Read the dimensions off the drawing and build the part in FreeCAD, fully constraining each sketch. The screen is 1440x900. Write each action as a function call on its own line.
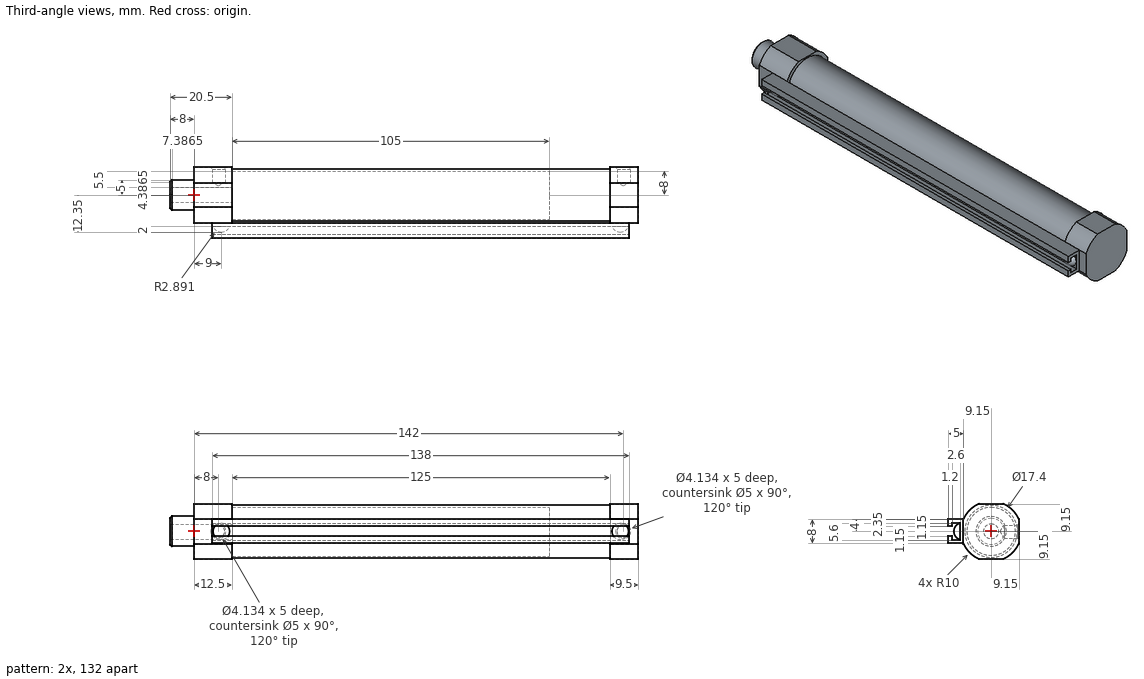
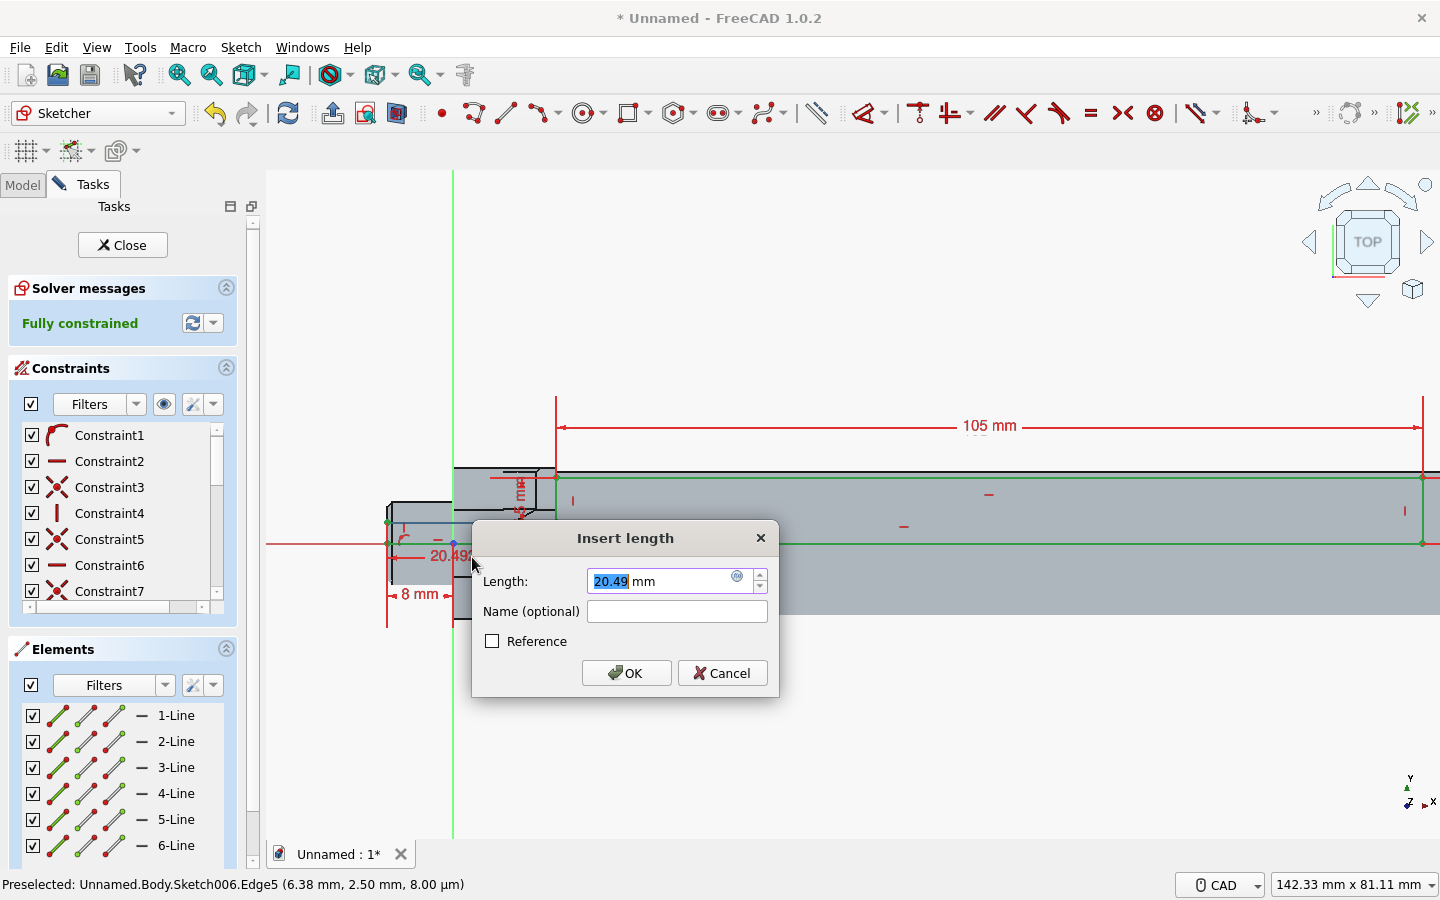
text(20.5)
key(Return)
key(Escape)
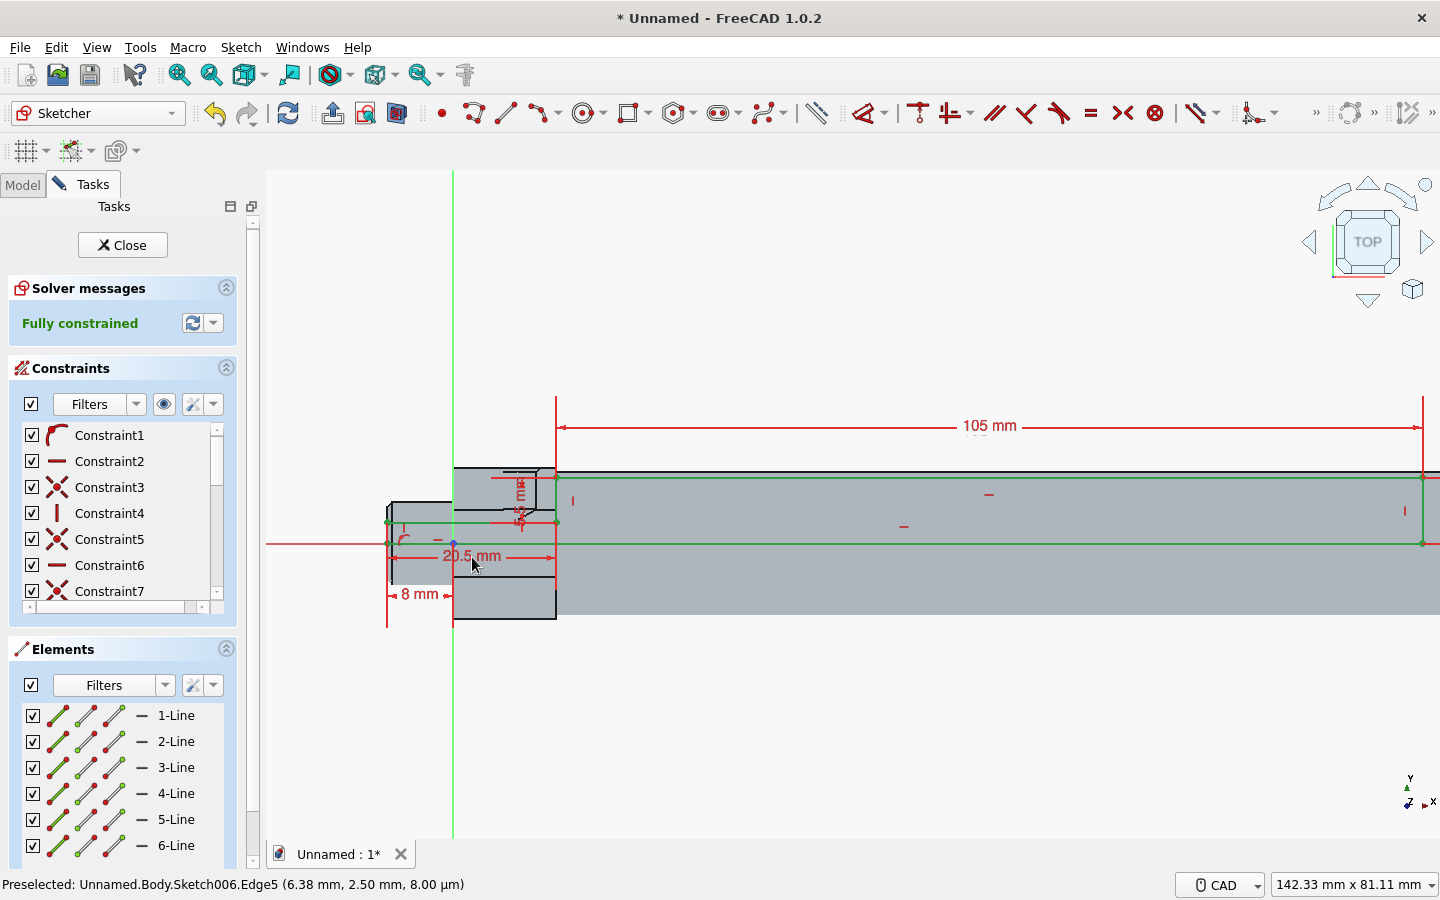
click(123, 245)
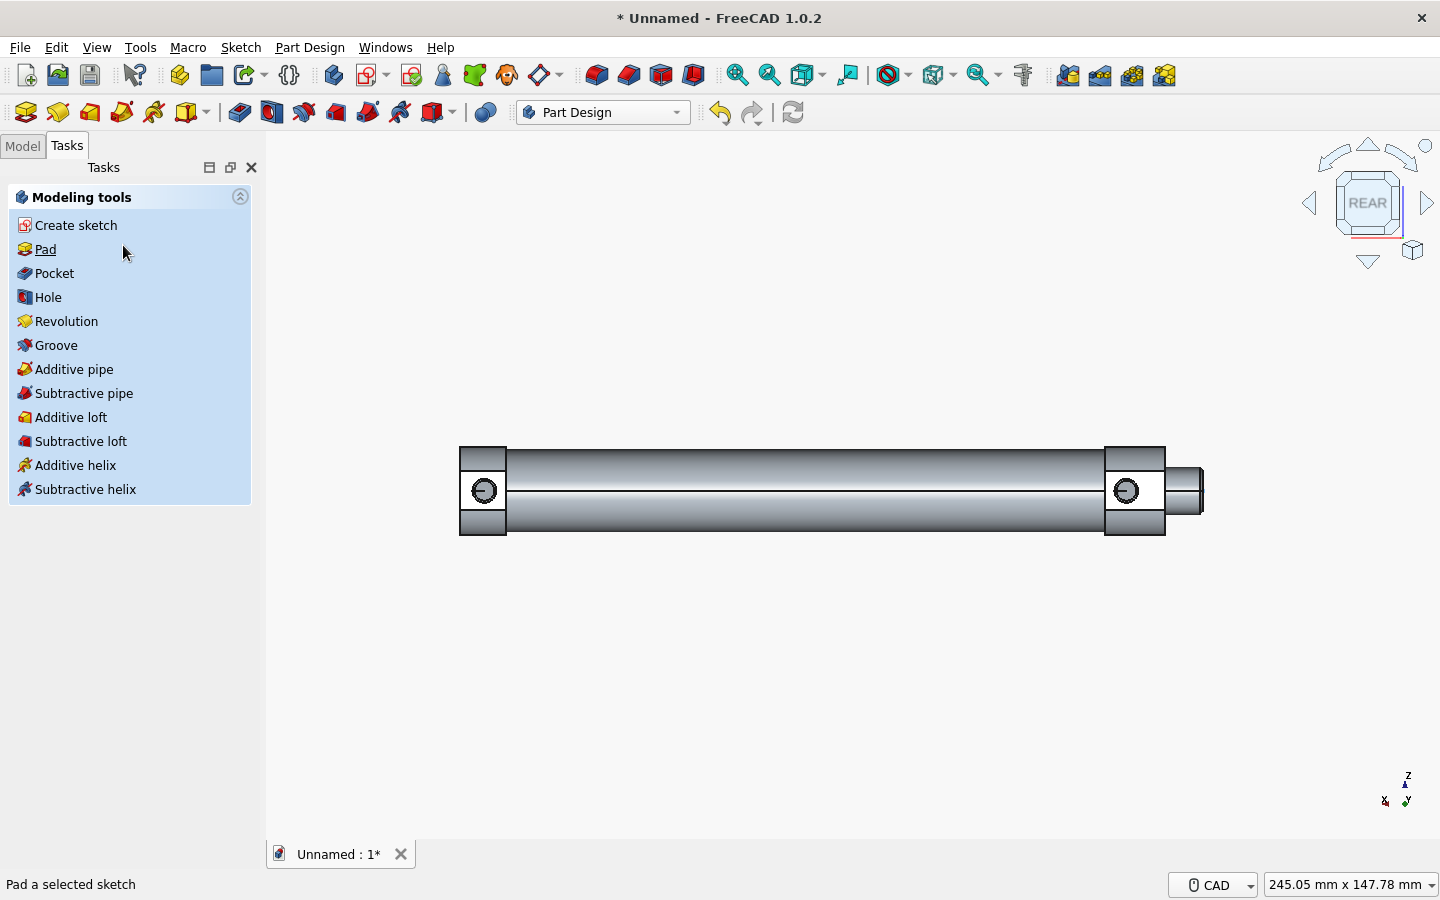
click(304, 112)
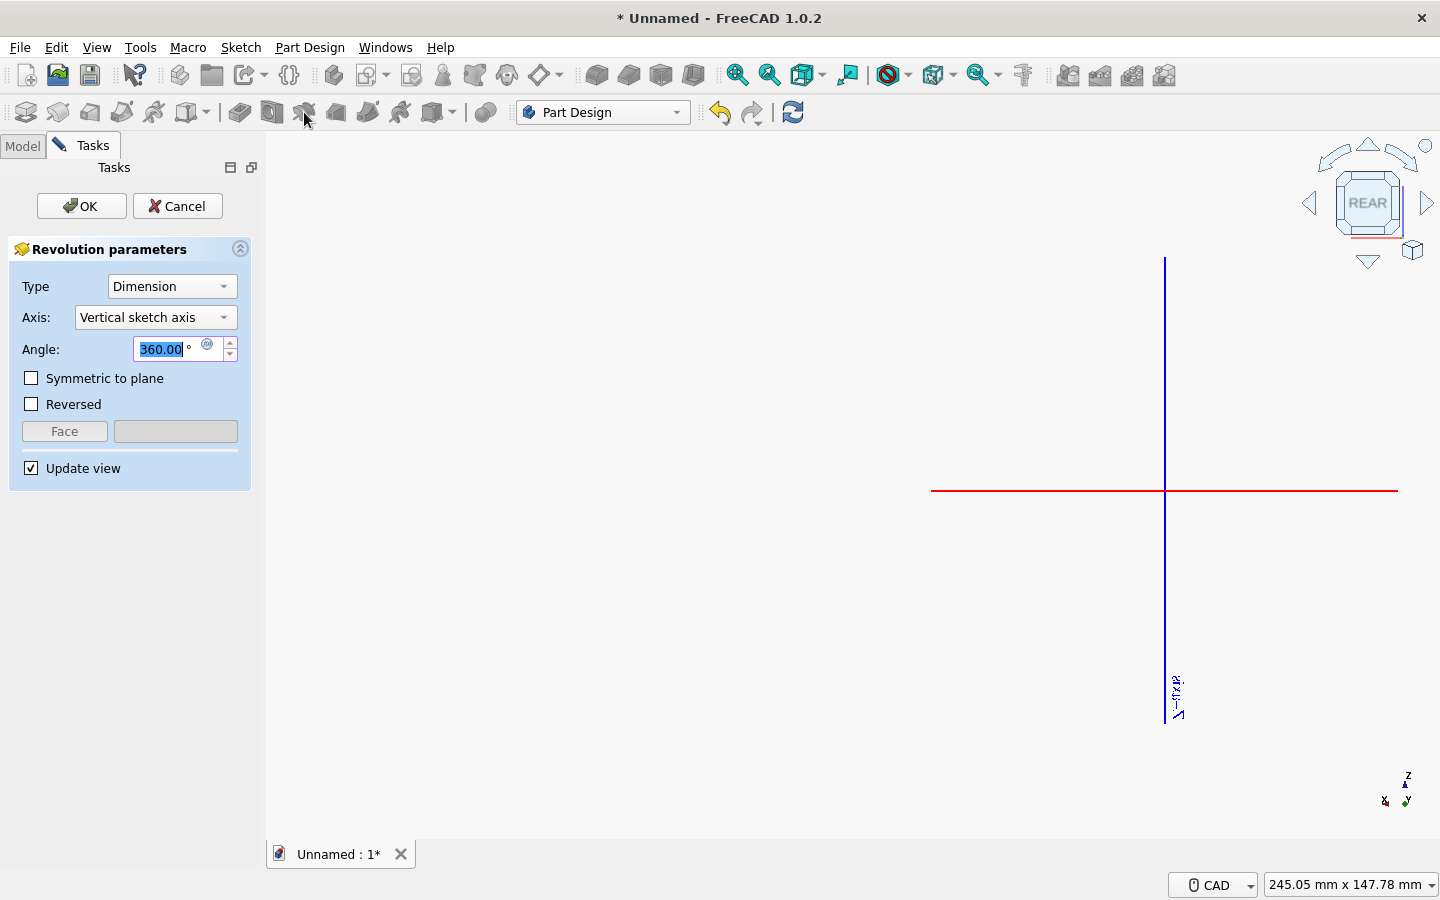
click(156, 318)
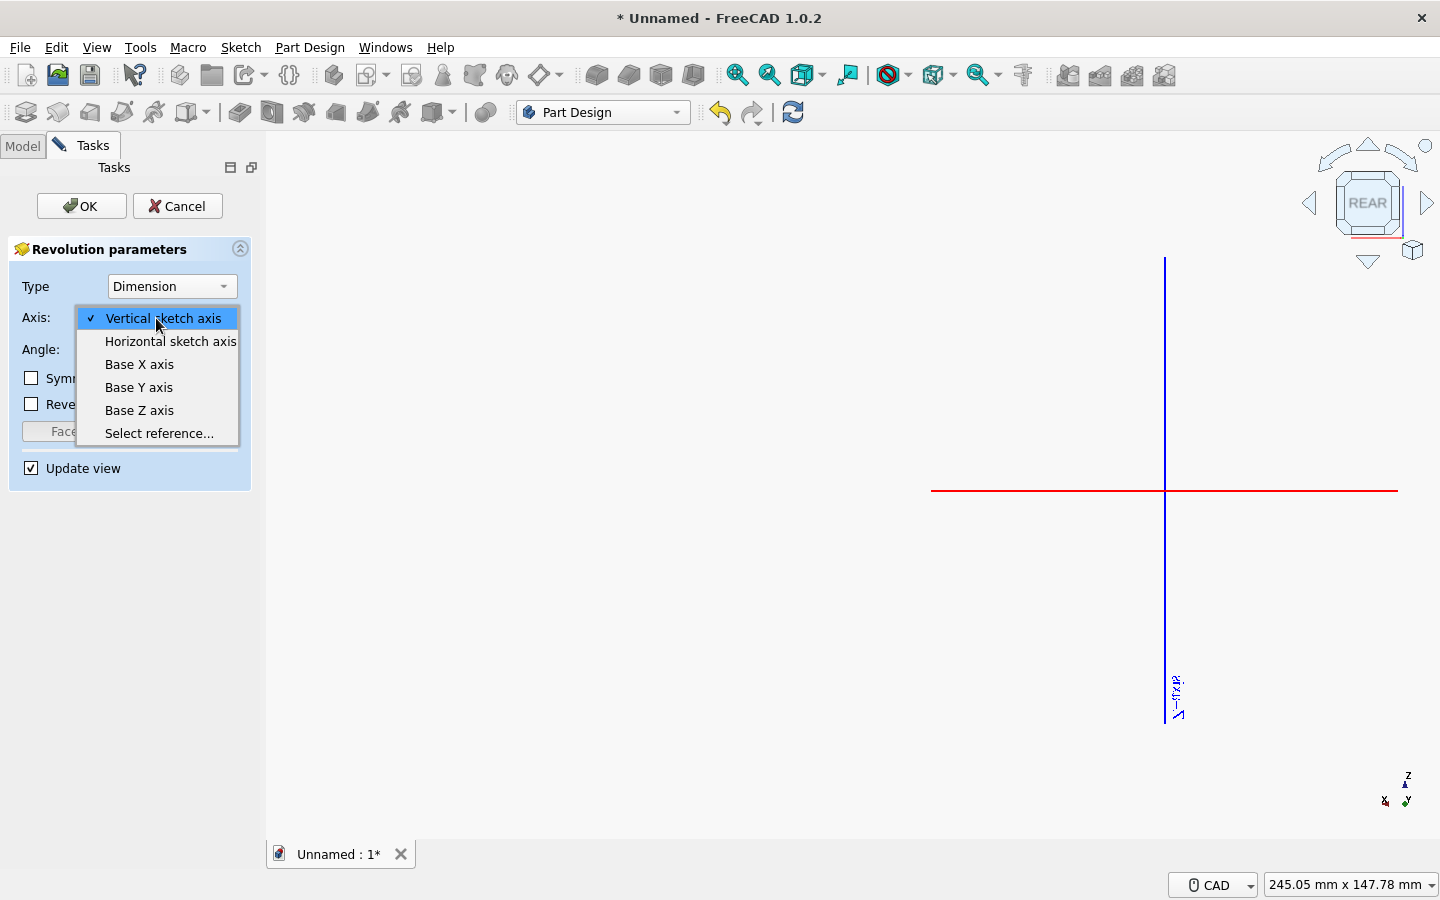
click(156, 342)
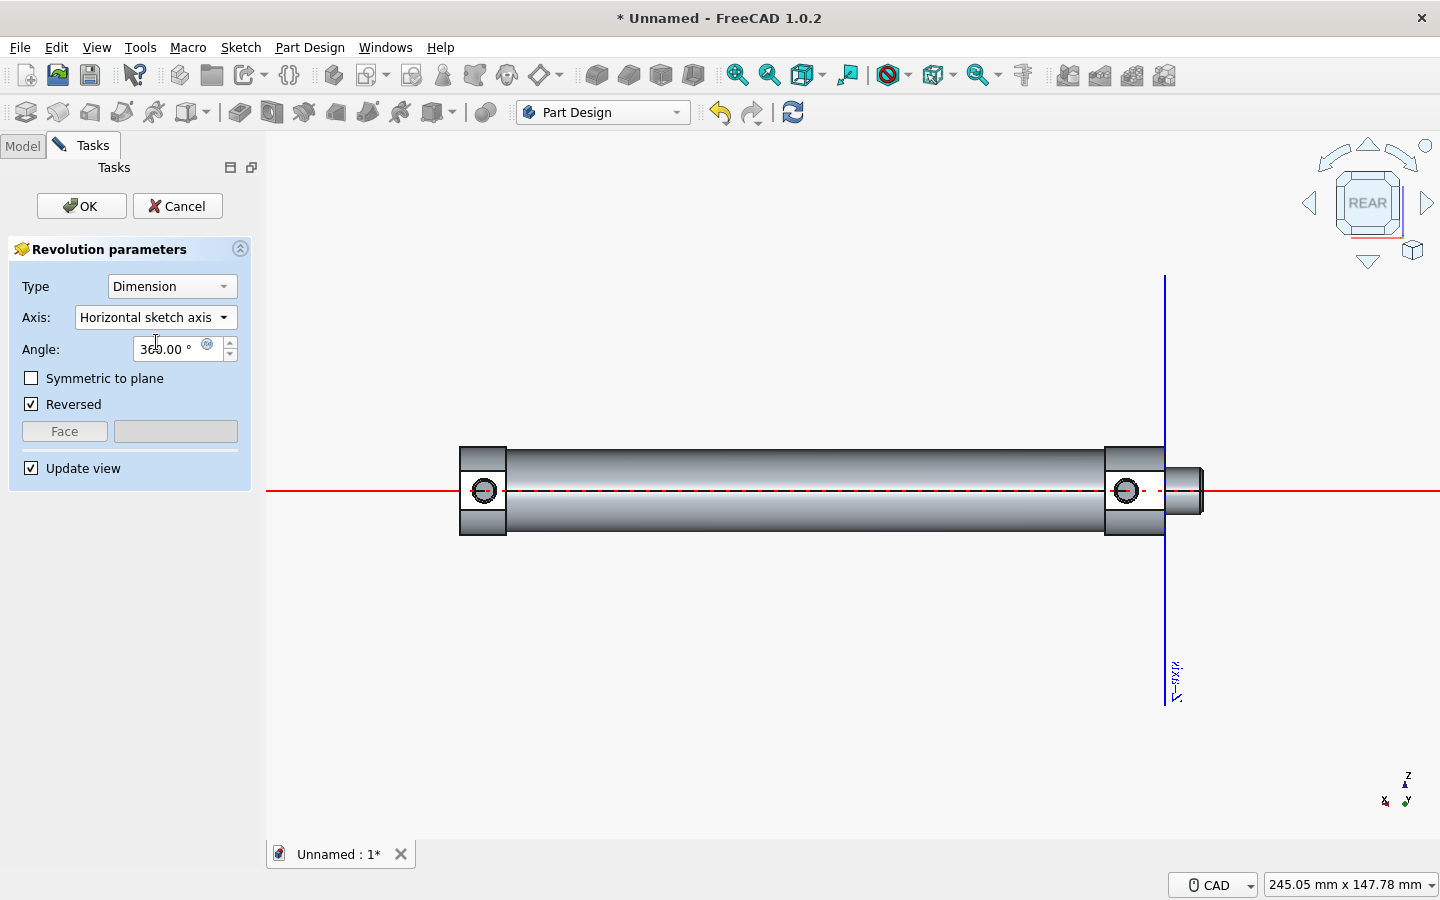
click(82, 206)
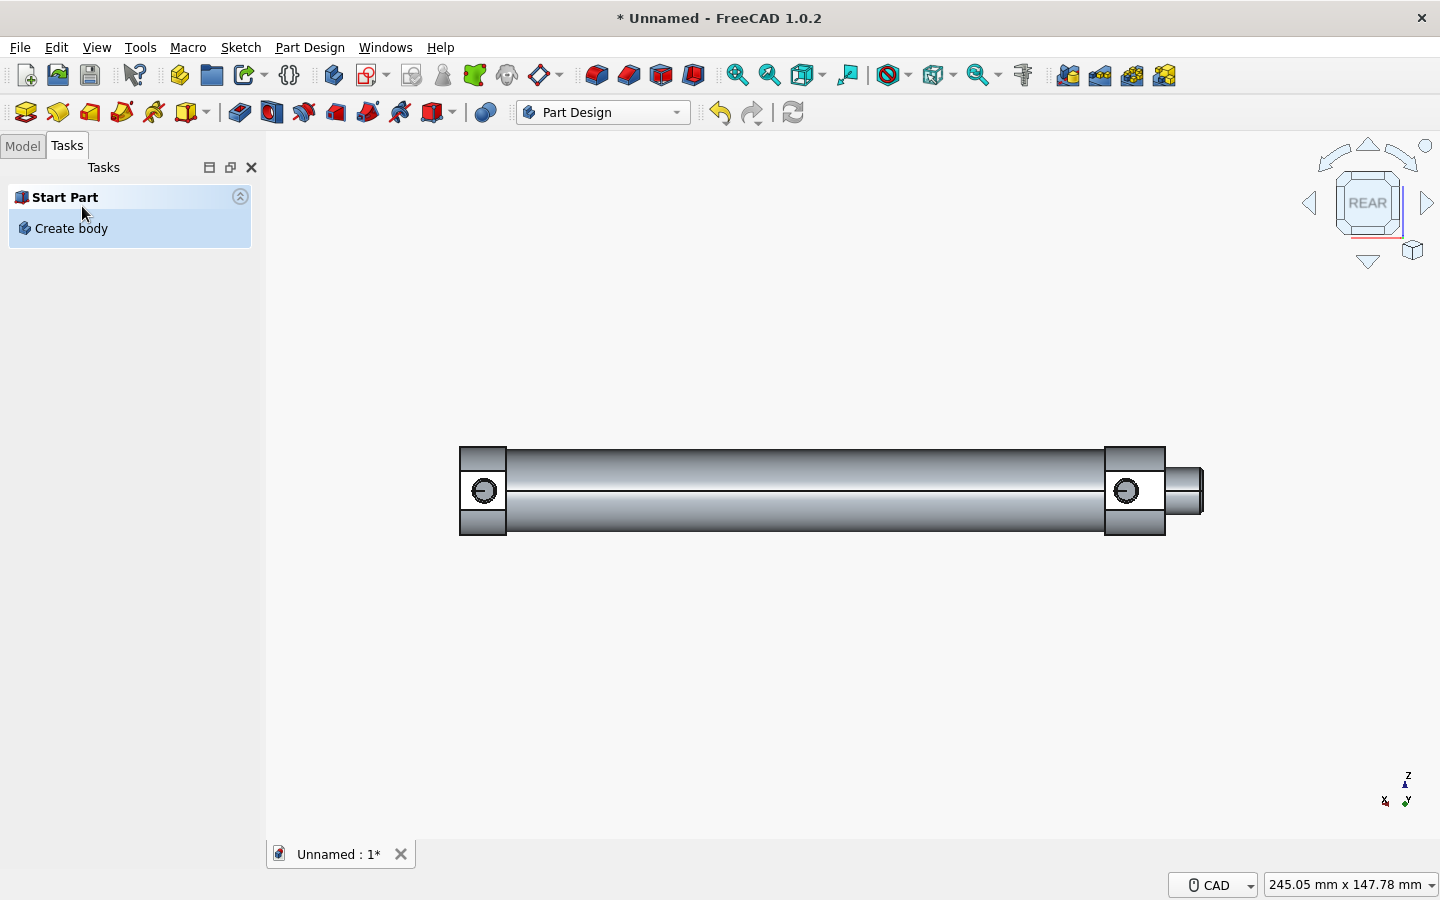
click(23, 145)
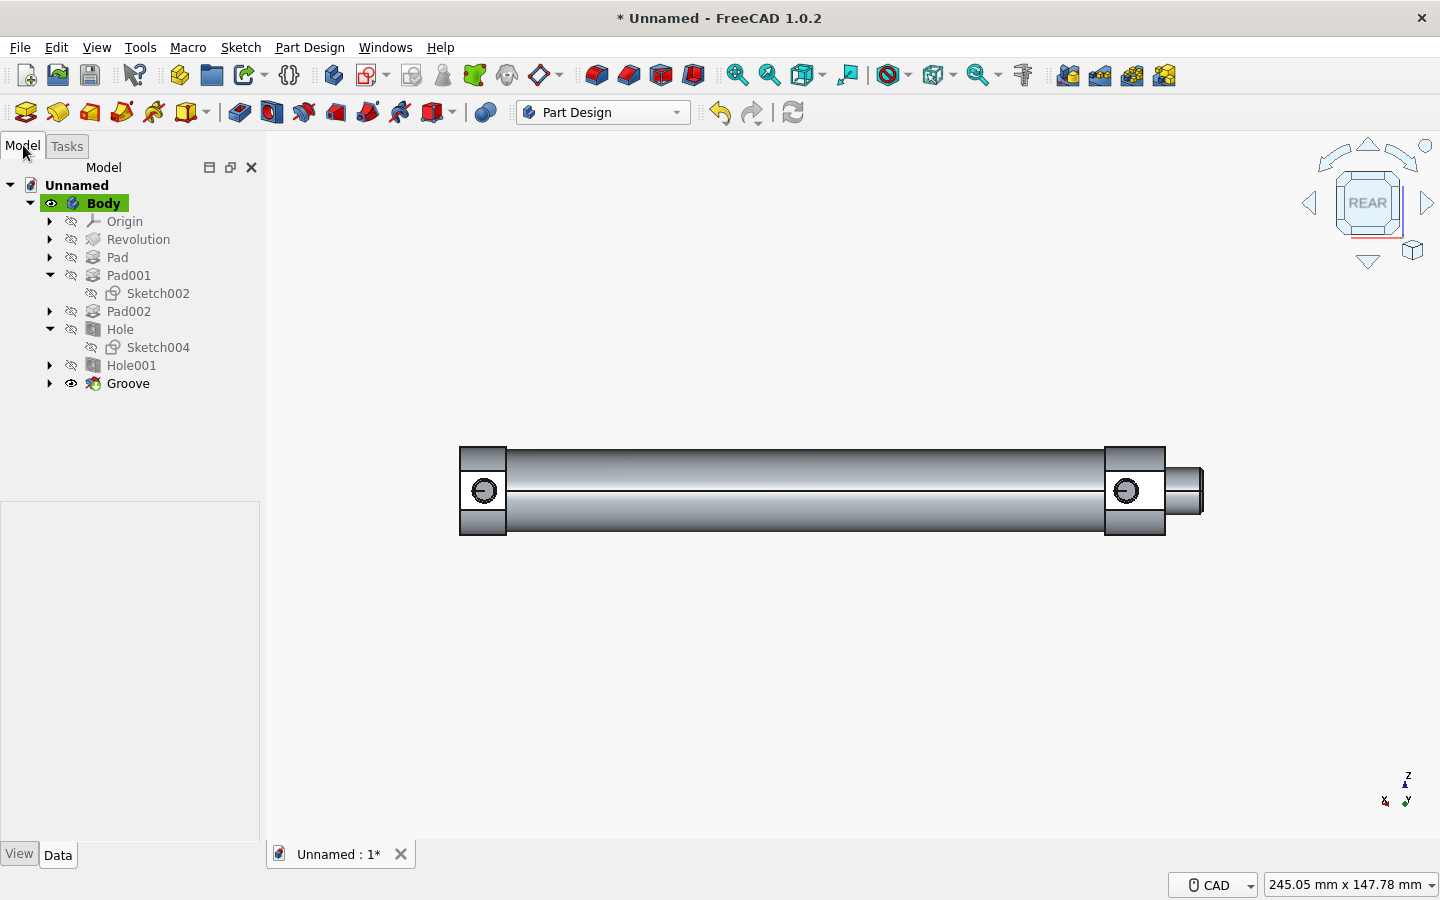
click(50, 221)